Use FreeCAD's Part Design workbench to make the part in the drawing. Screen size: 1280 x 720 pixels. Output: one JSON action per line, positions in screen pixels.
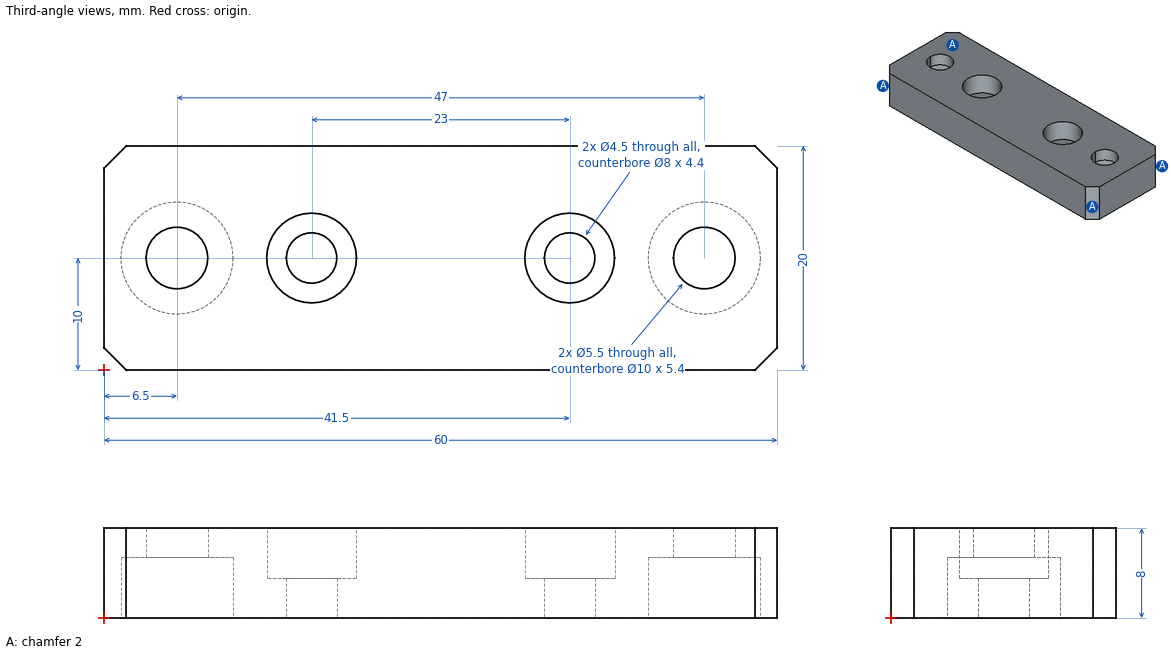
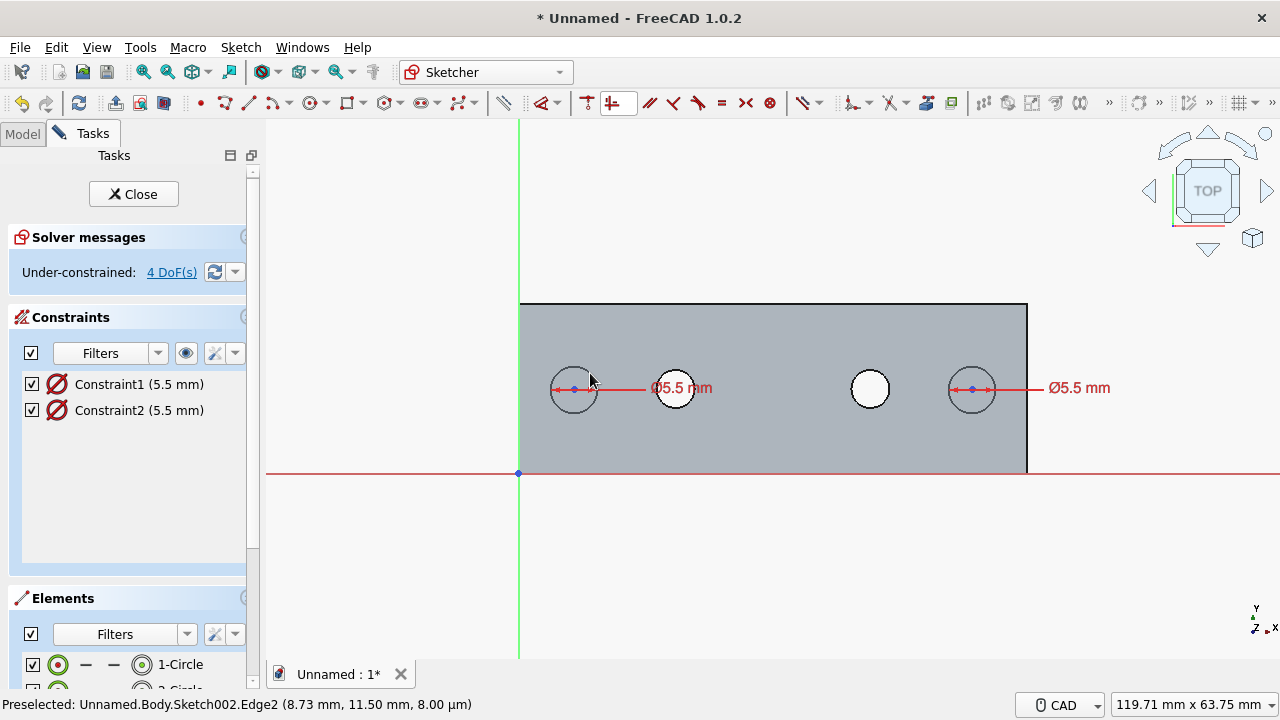
{"action": "left_click", "coordinate": [972, 390]}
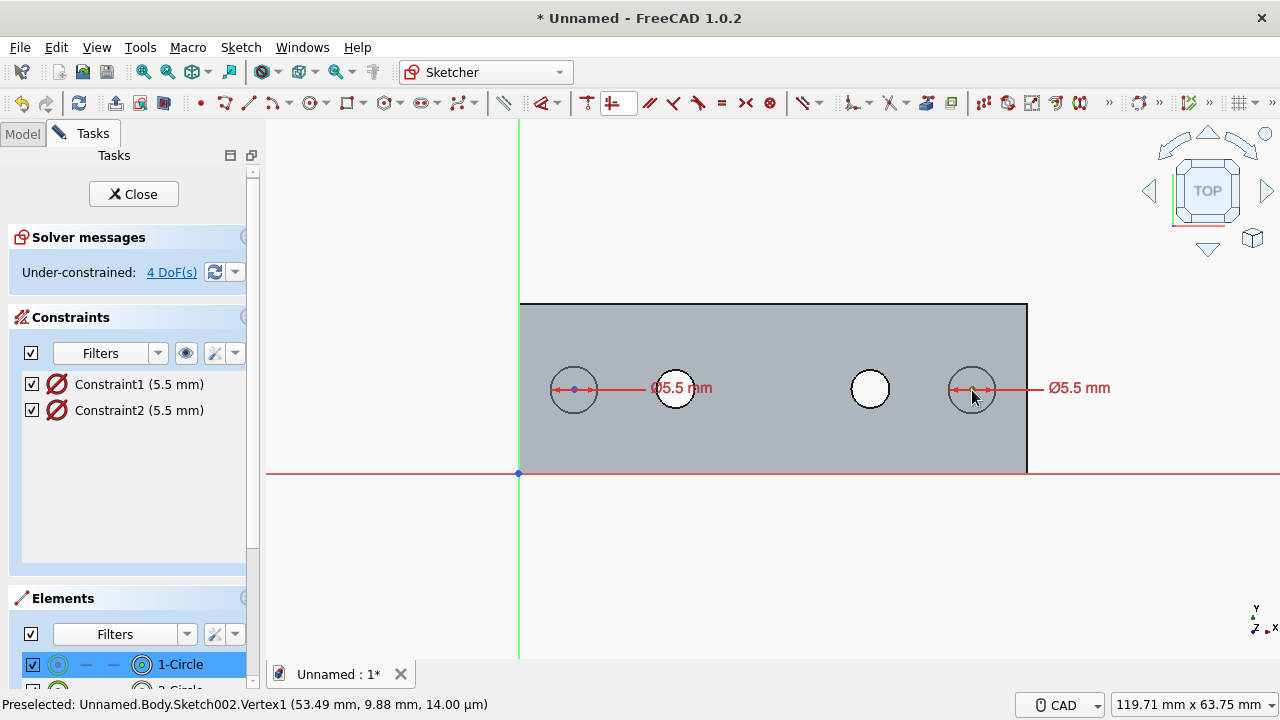
{"action": "left_click", "coordinate": [574, 390]}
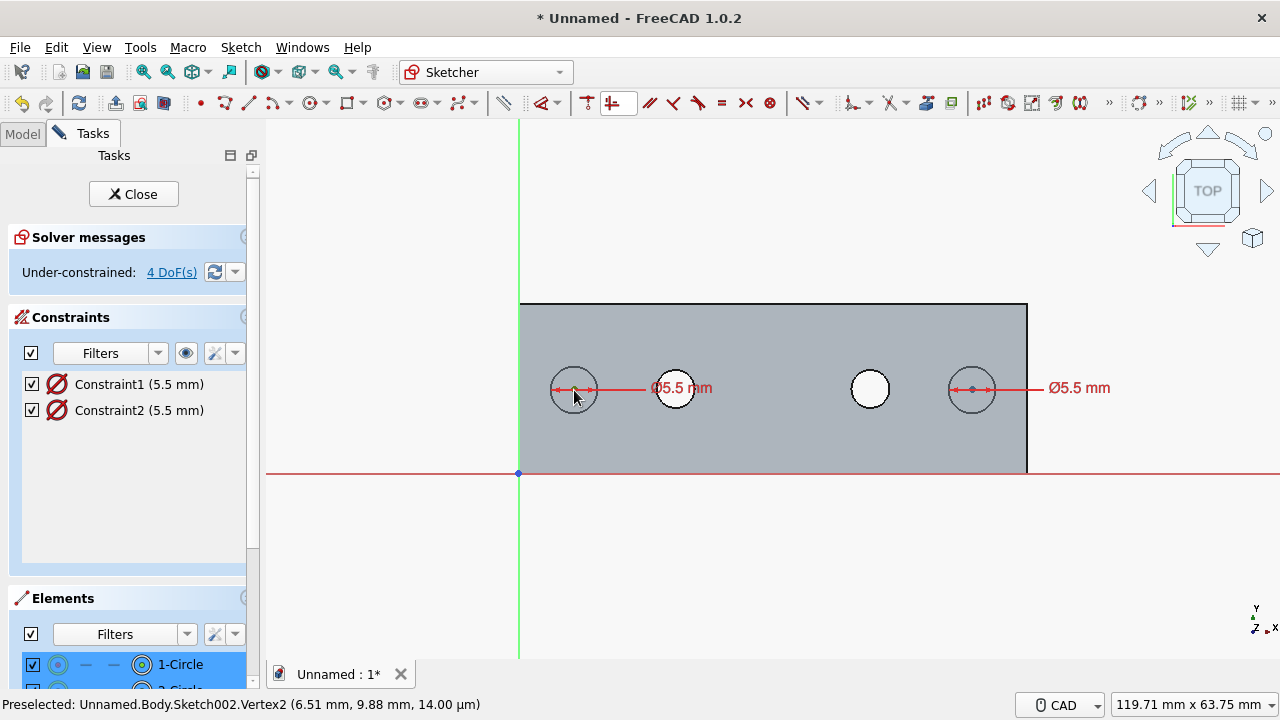
{"action": "key", "text": "h"}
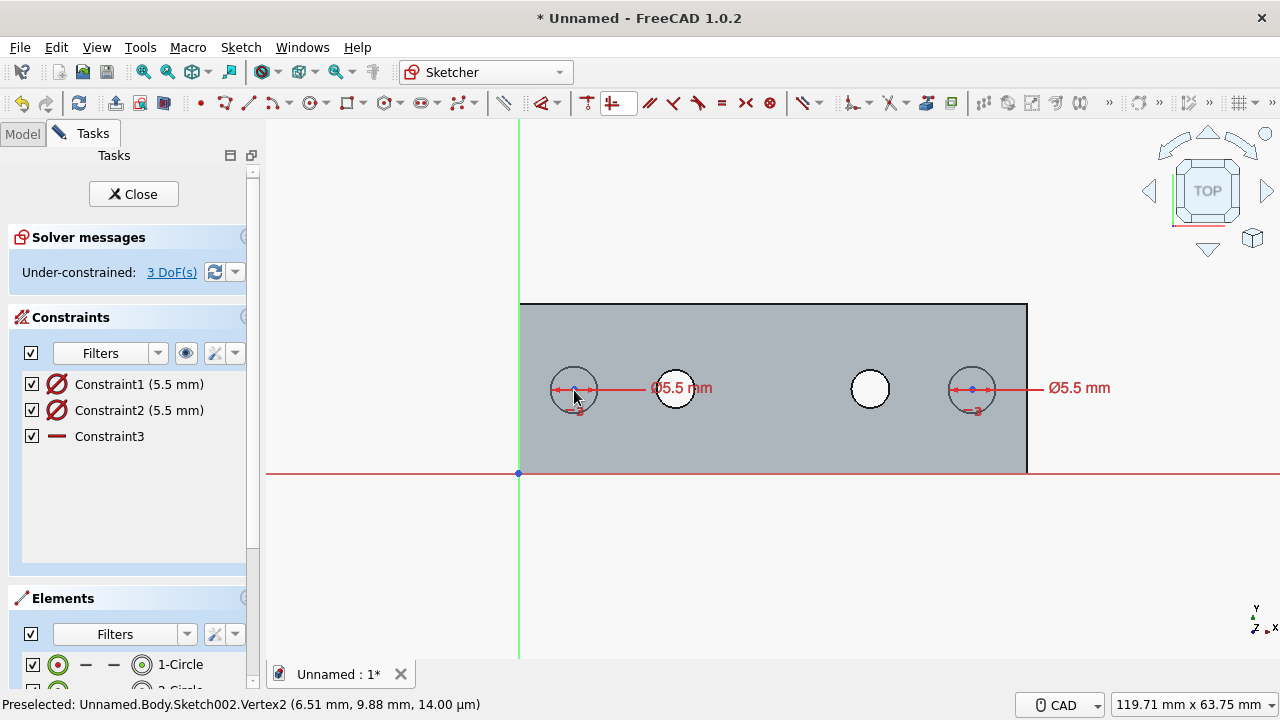
{"action": "key", "text": "d"}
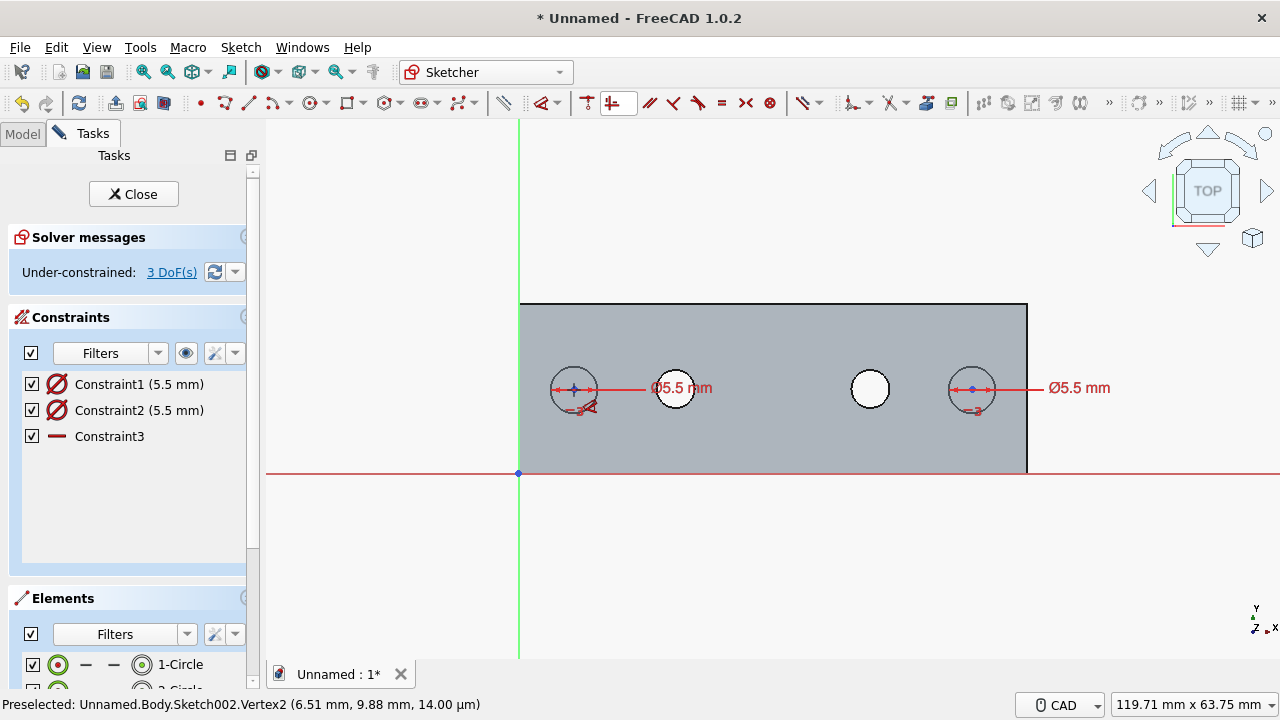
{"action": "left_click", "coordinate": [972, 390]}
{"action": "left_click", "coordinate": [485, 432]}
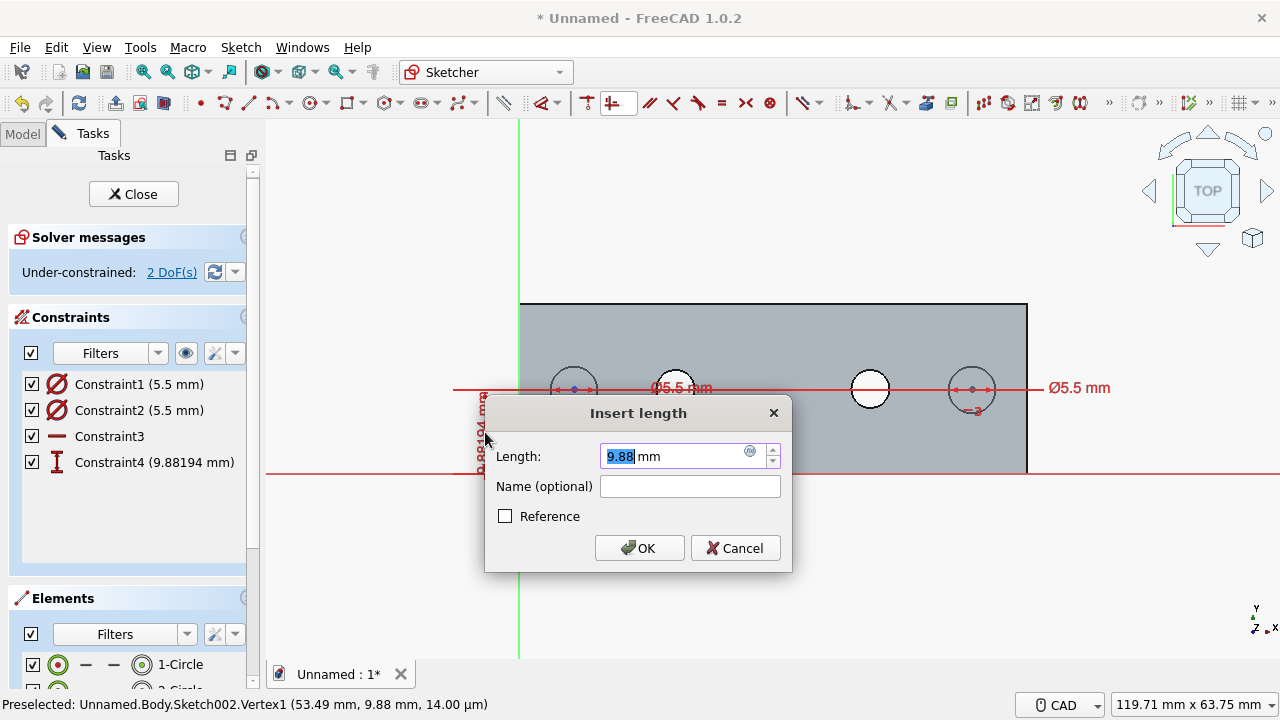
{"action": "type", "text": "10"}
{"action": "key", "text": "Return"}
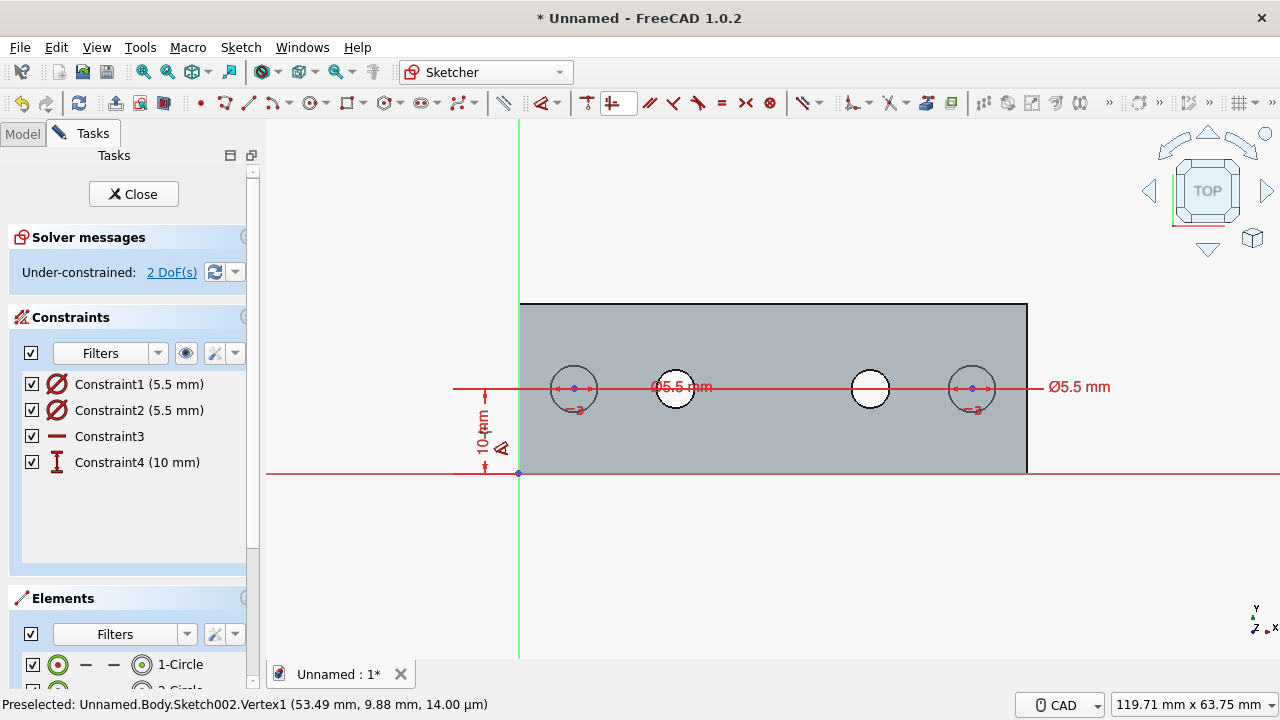
{"action": "left_click", "coordinate": [574, 389]}
{"action": "left_click", "coordinate": [546, 508]}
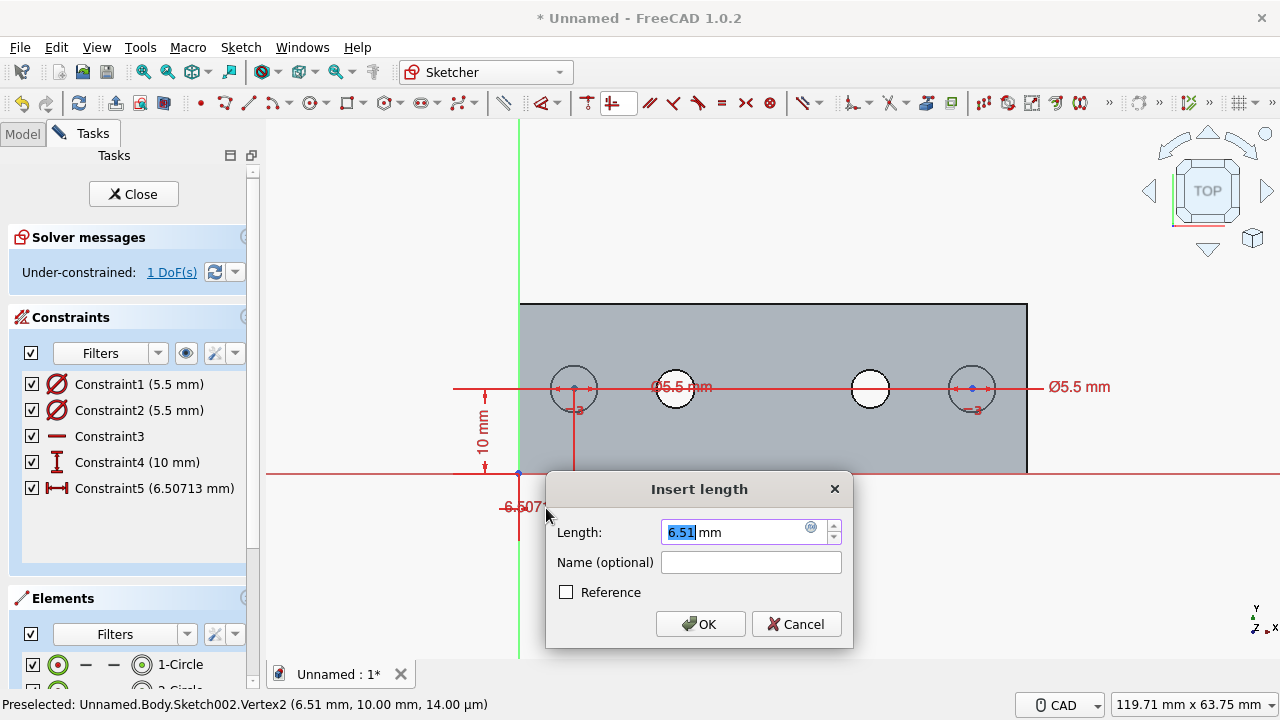
{"action": "type", "text": "6.5"}
{"action": "key", "text": "Return"}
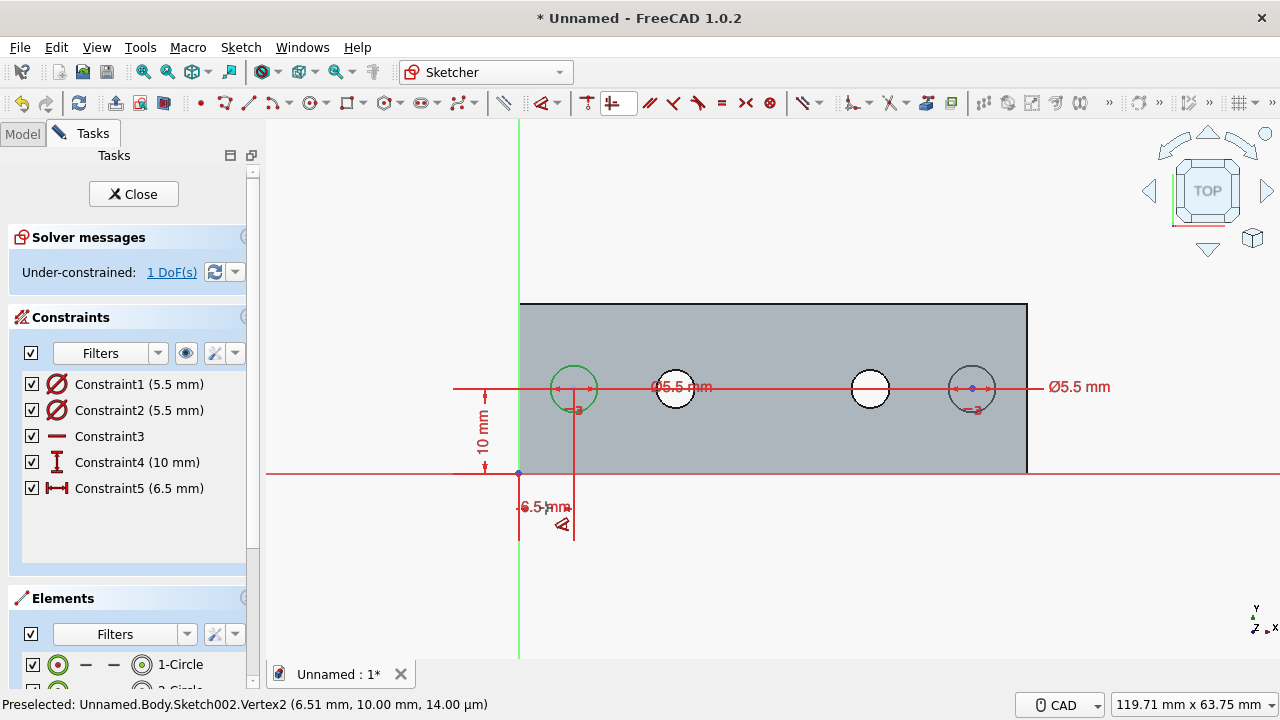
{"action": "left_click", "coordinate": [972, 389]}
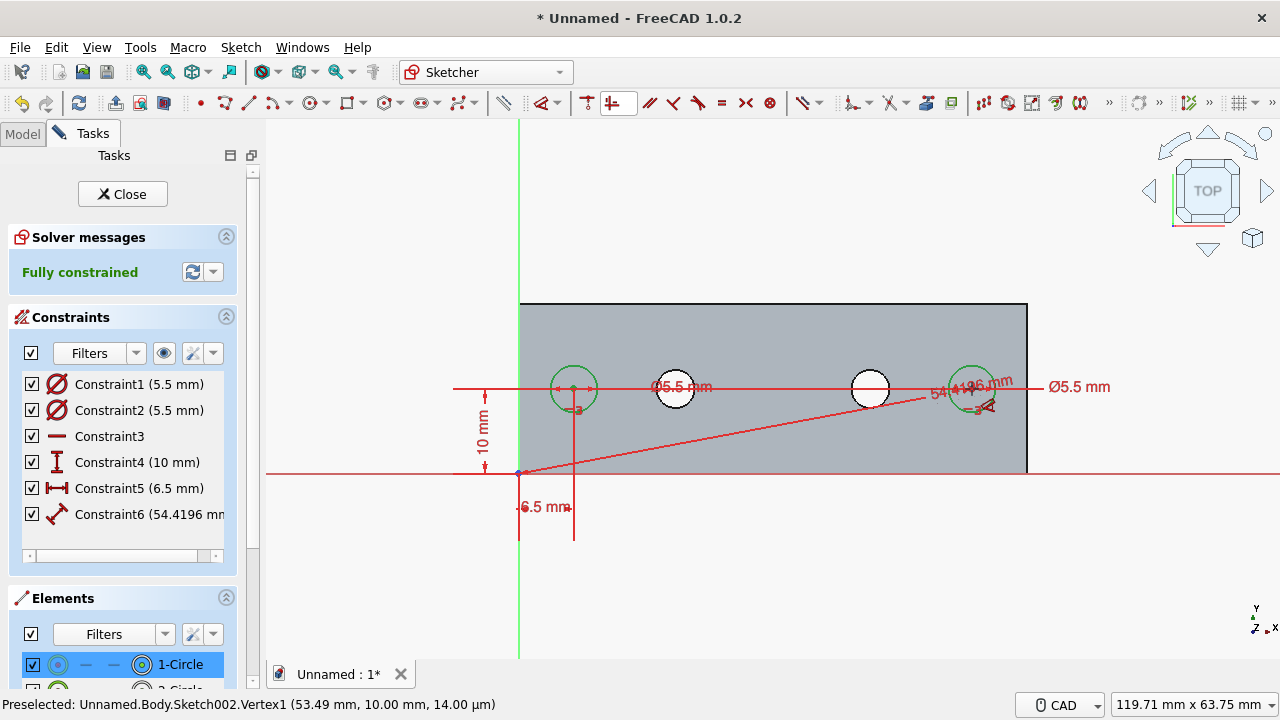
{"action": "left_click", "coordinate": [574, 389]}
{"action": "left_click", "coordinate": [773, 355]}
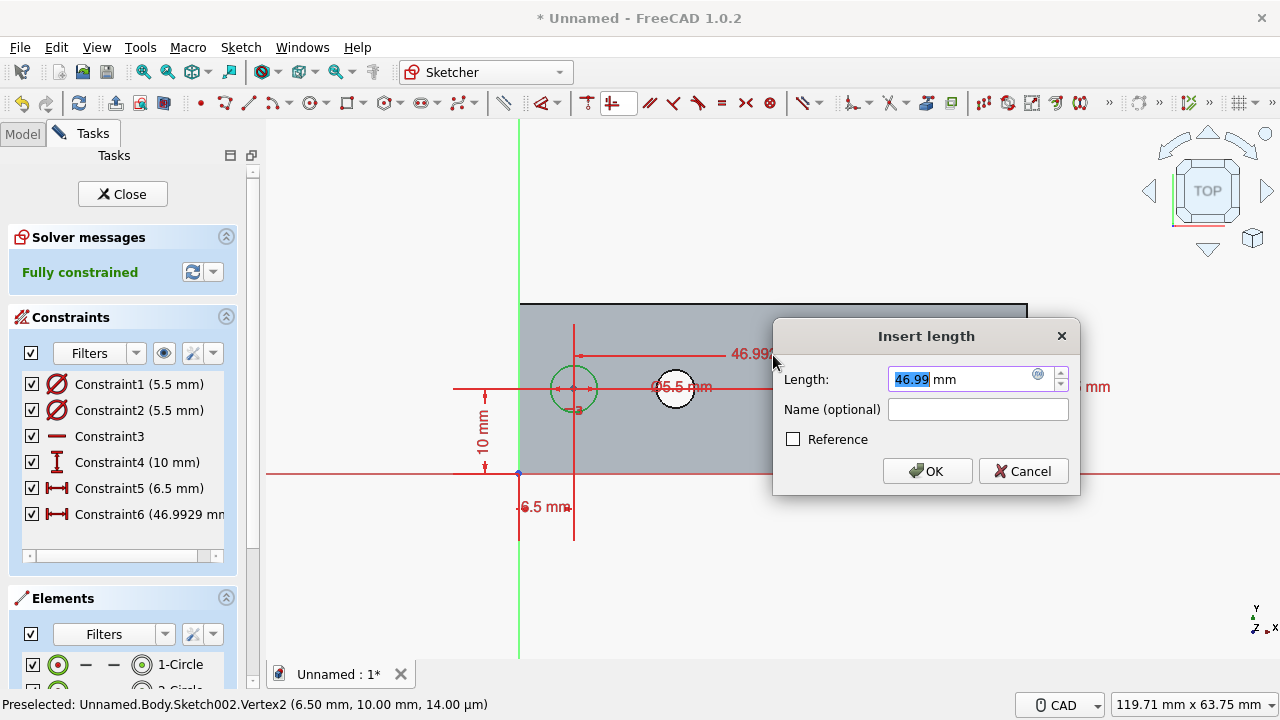
{"action": "type", "text": "47"}
{"action": "key", "text": "Return"}
{"action": "key", "text": "Escape"}